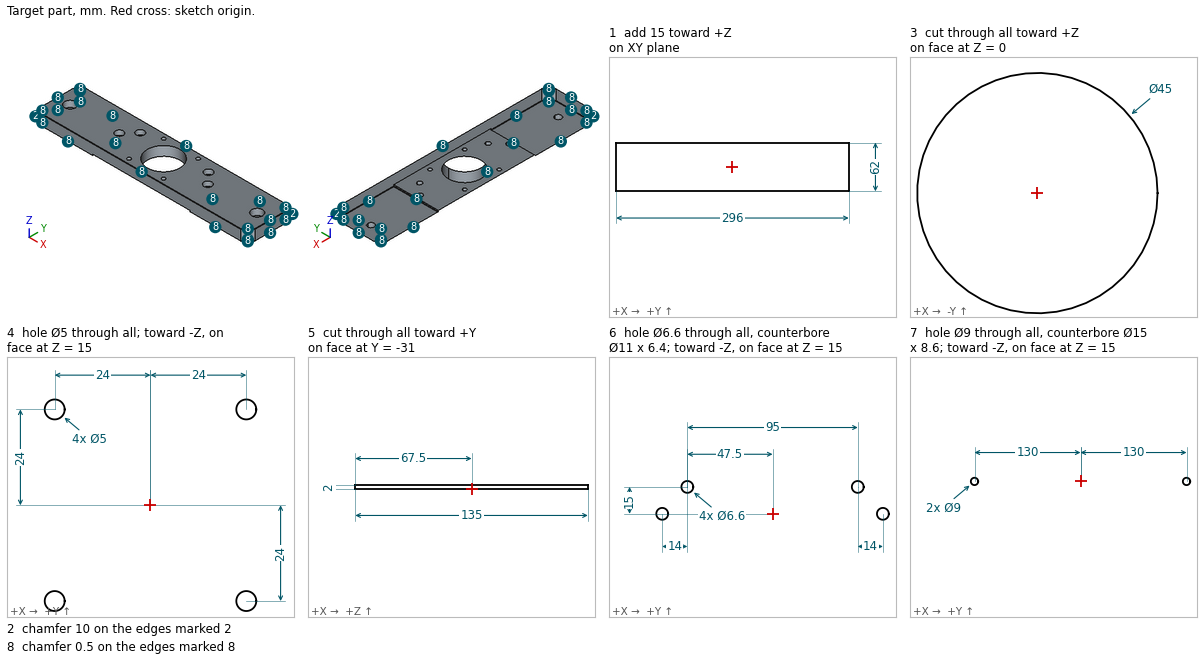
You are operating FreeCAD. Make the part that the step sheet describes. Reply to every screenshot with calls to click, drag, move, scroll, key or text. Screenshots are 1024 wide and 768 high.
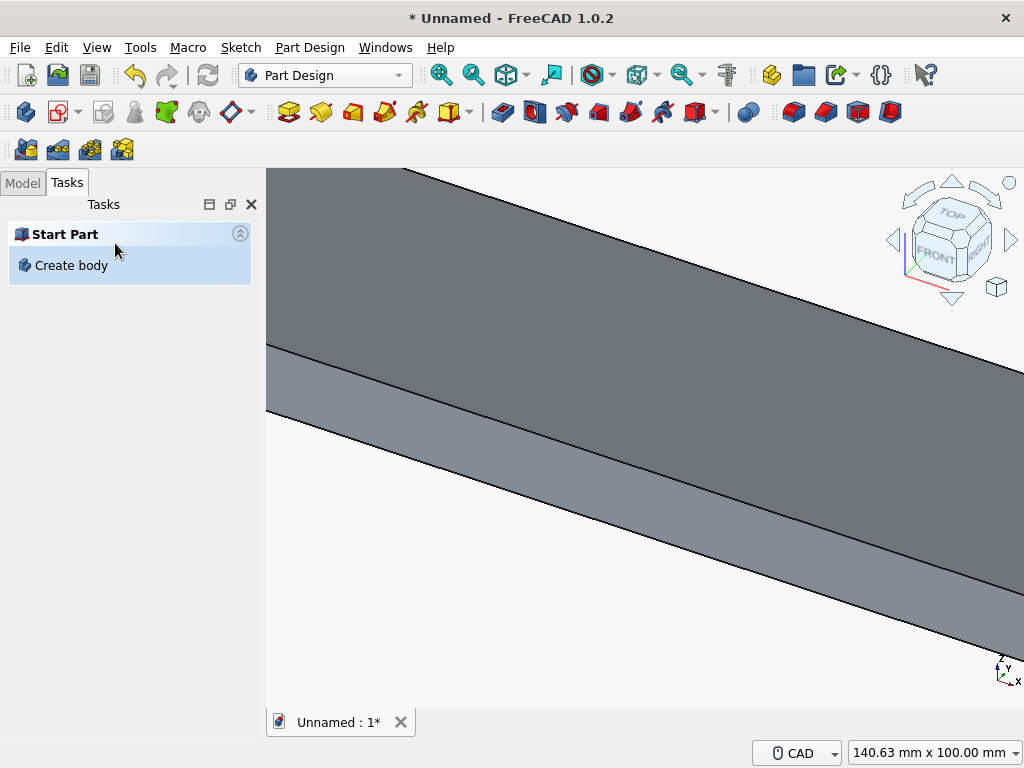
click(442, 76)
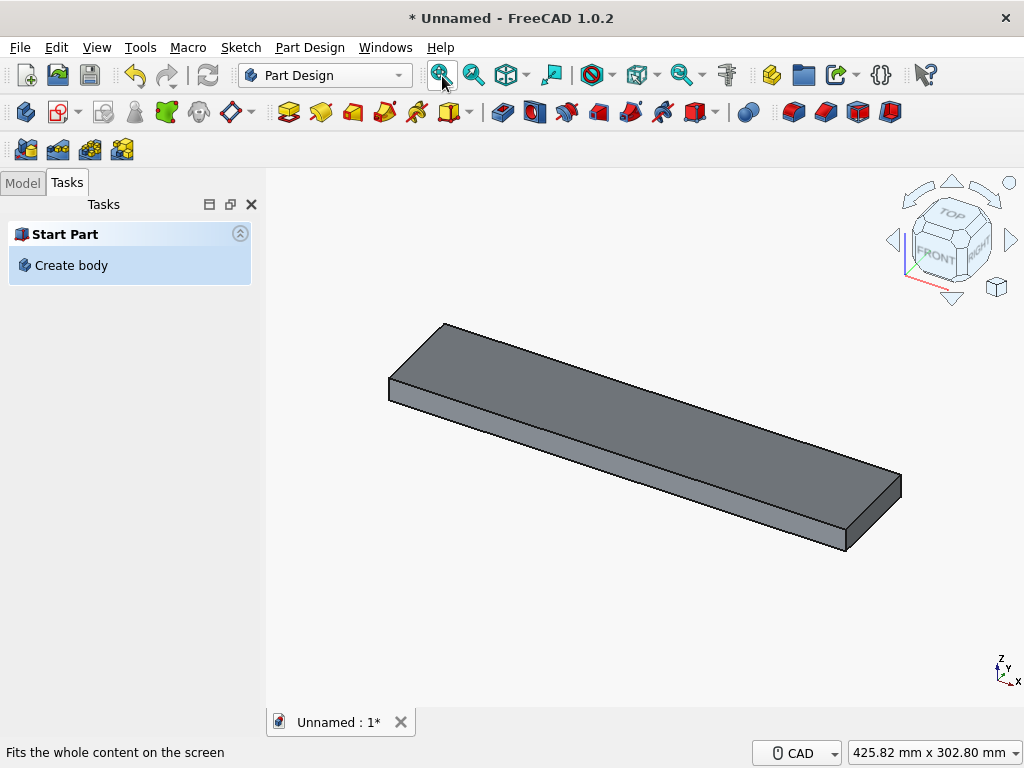
click(846, 539)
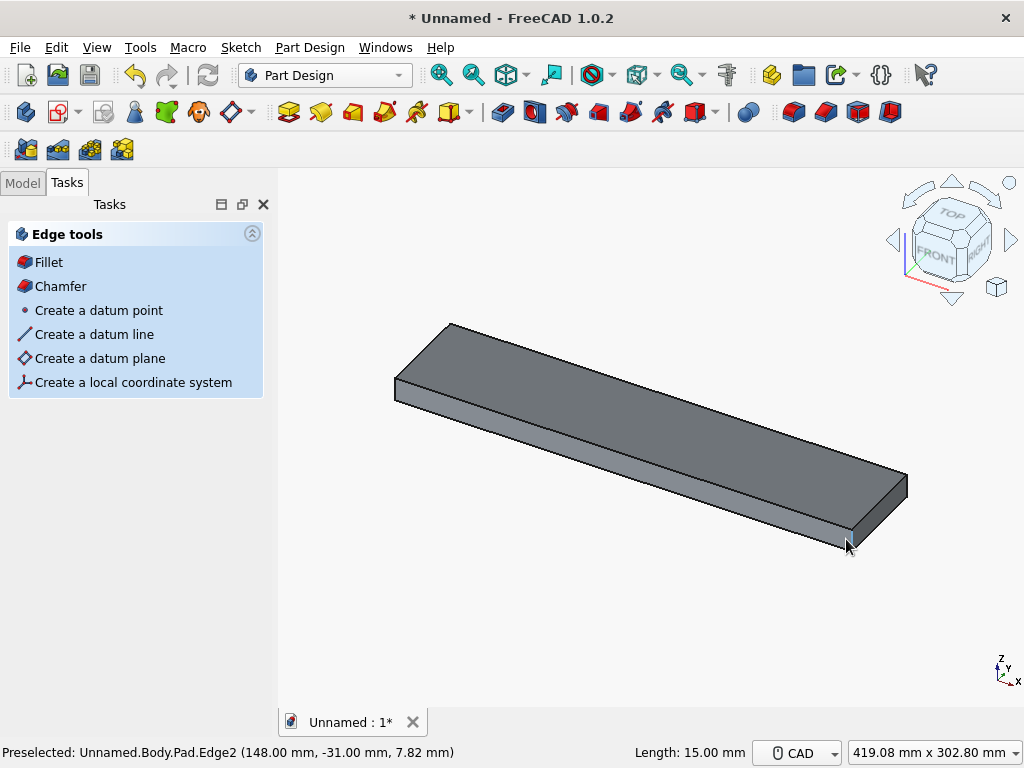
key(0)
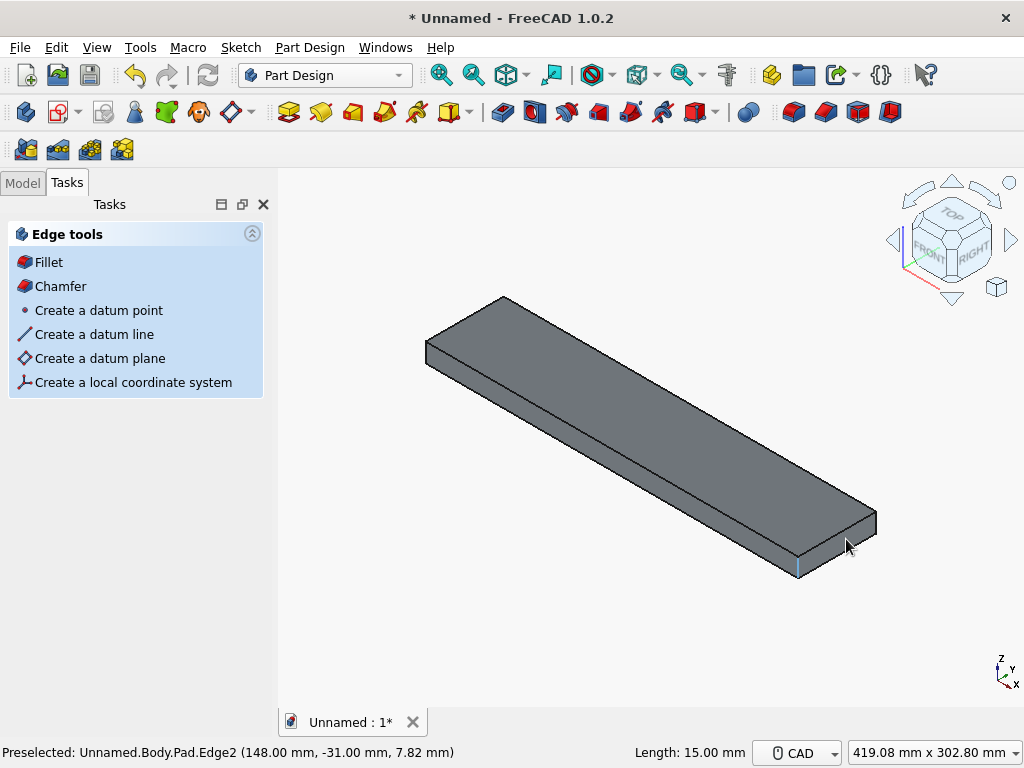
key(2)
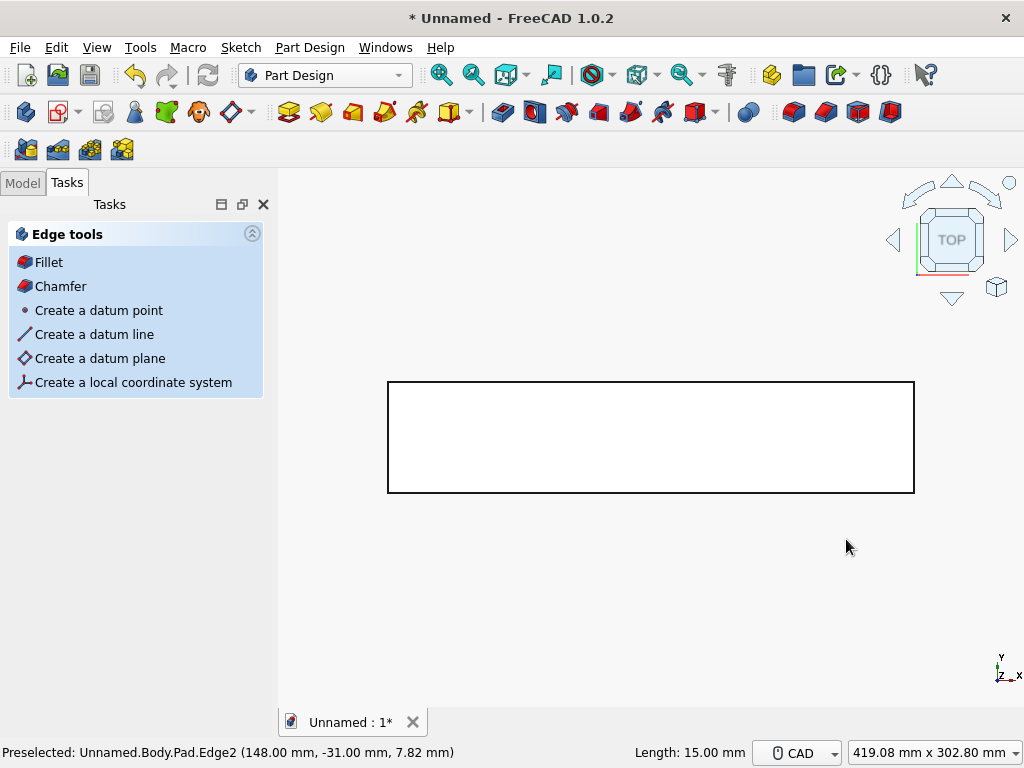
key(1)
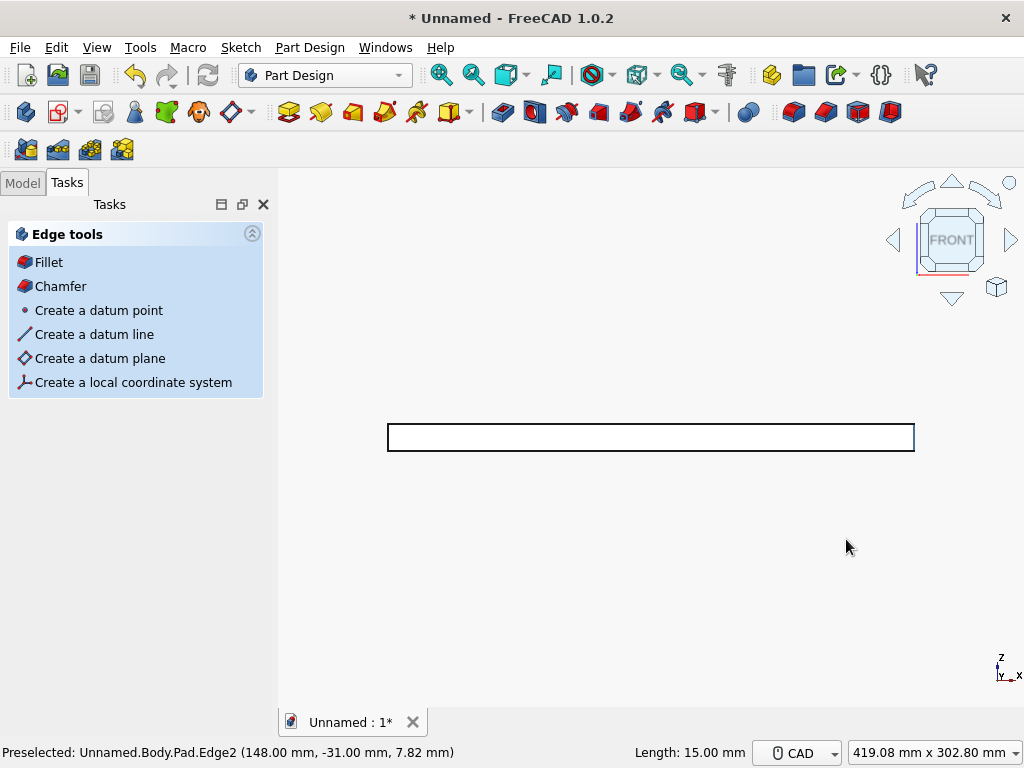
click(388, 436, ctrl)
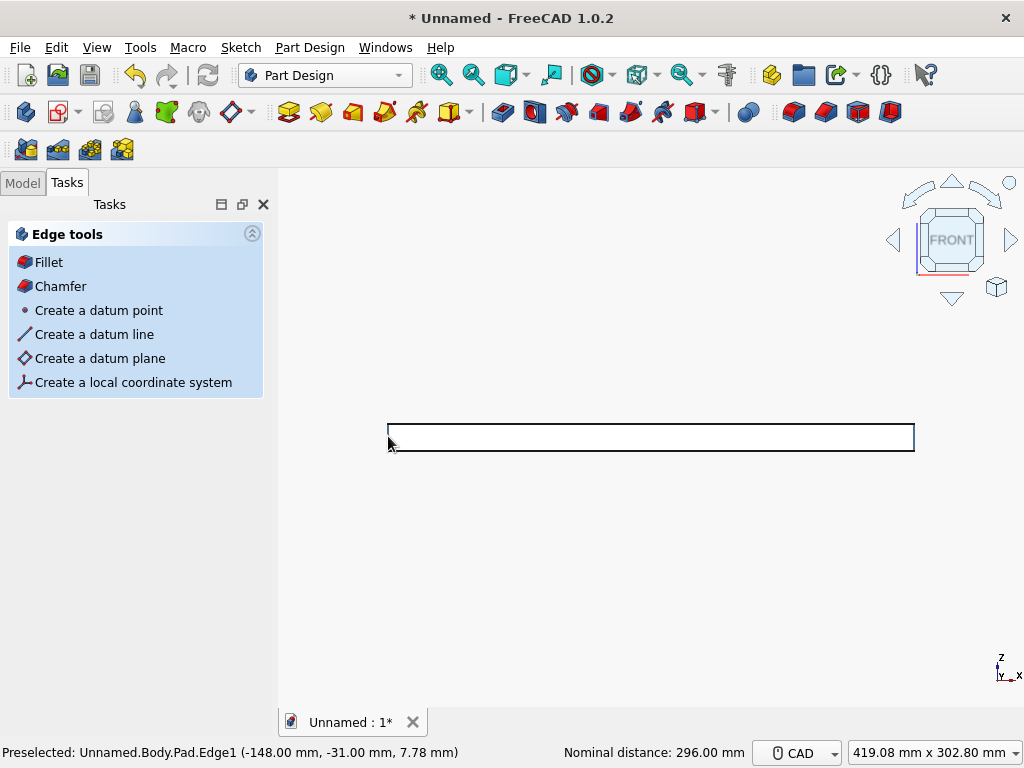
key(3)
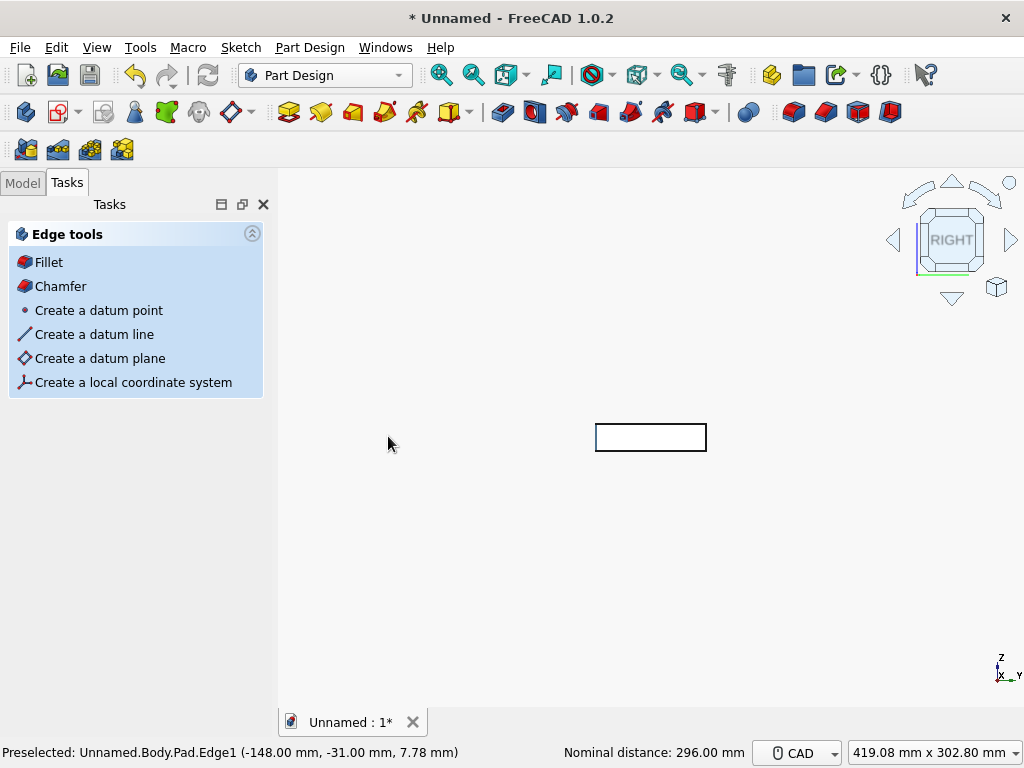
click(442, 76)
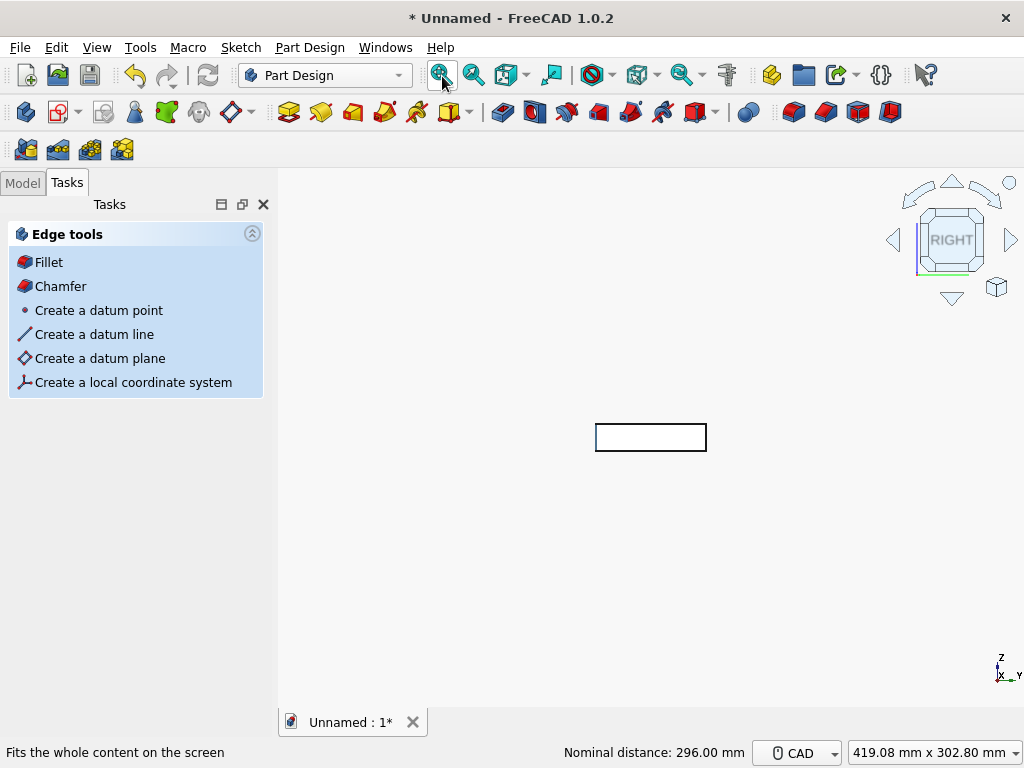
click(706, 436, ctrl)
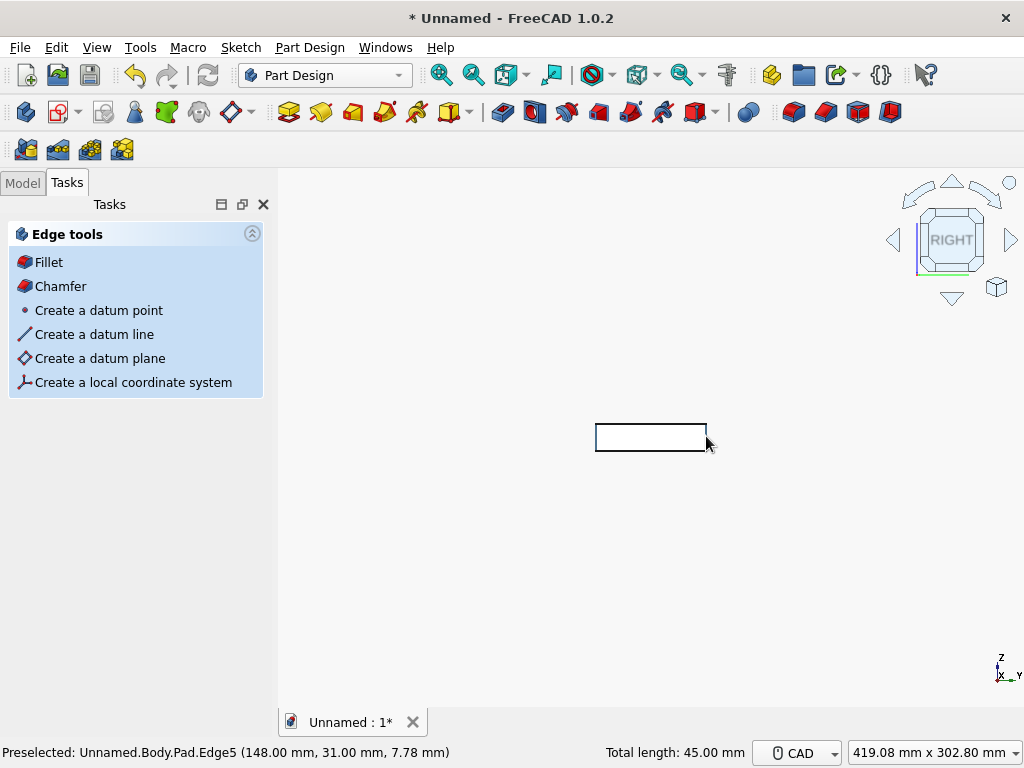
key(5)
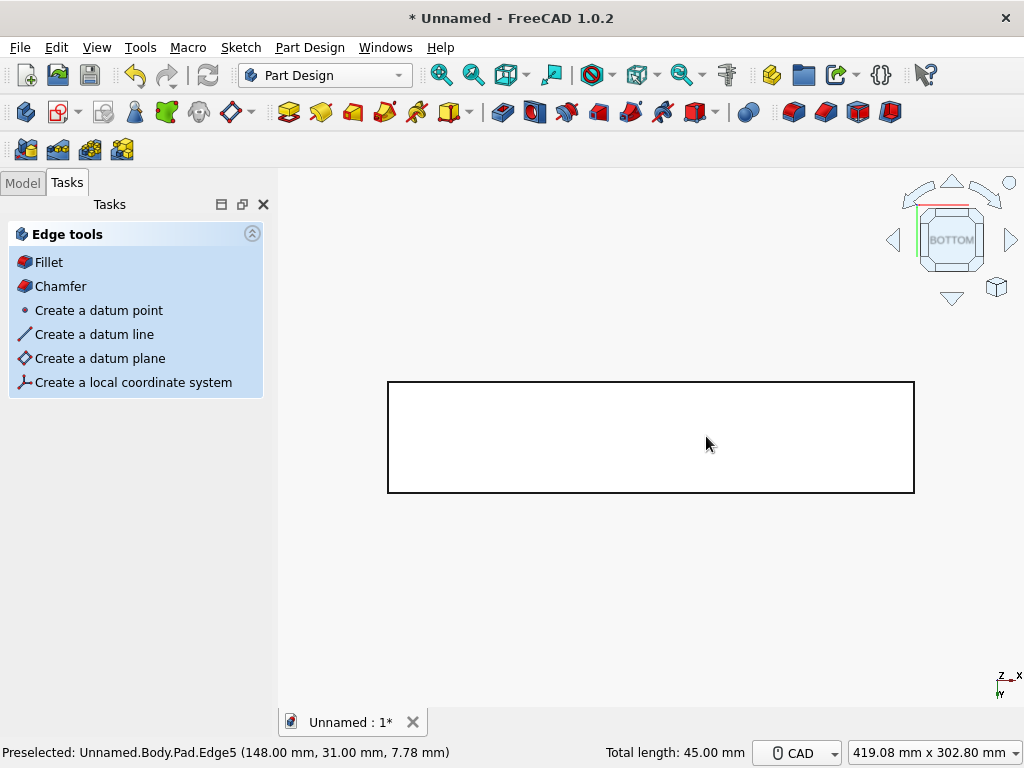
key(4)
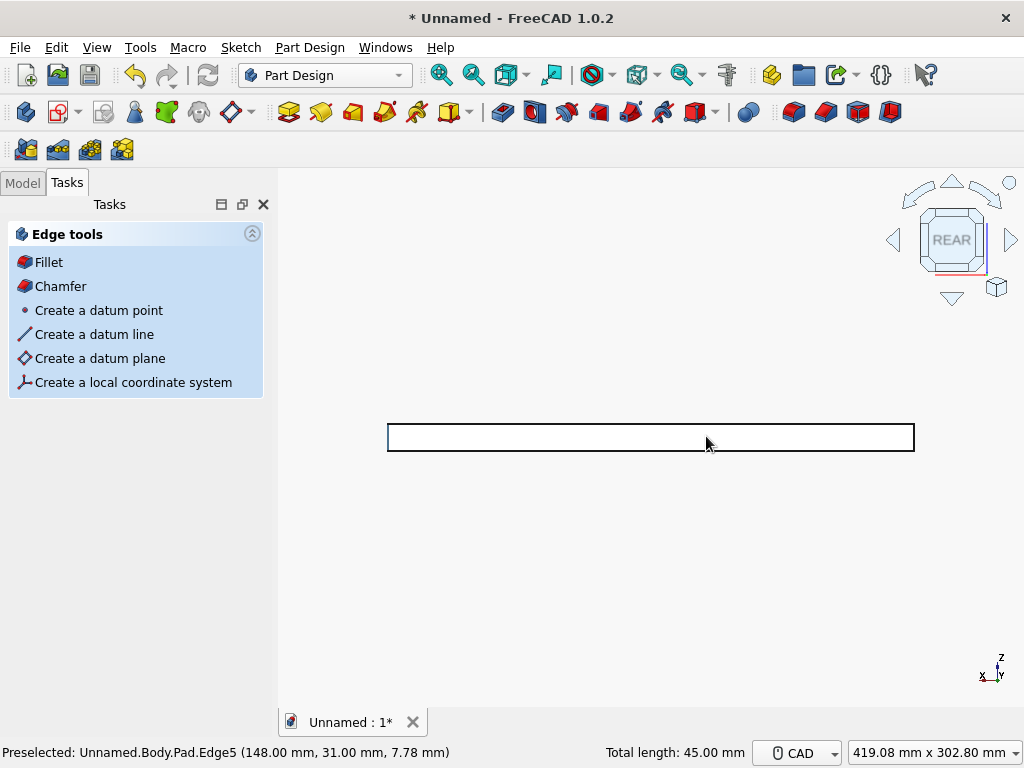
click(914, 437, ctrl)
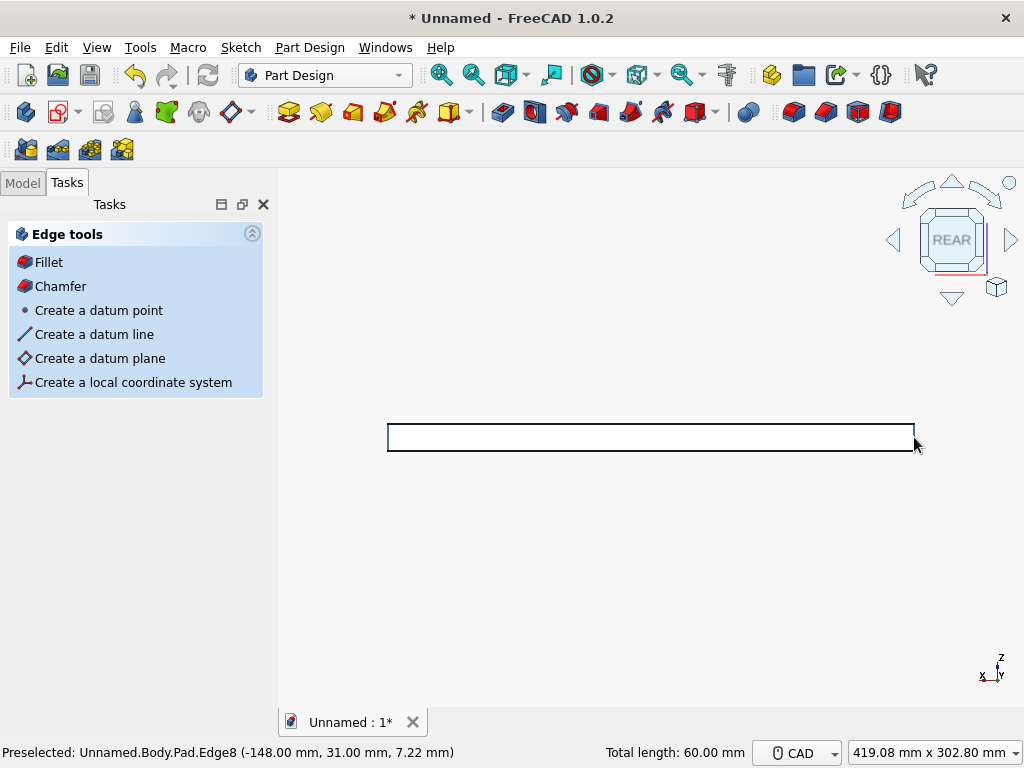
click(826, 112)